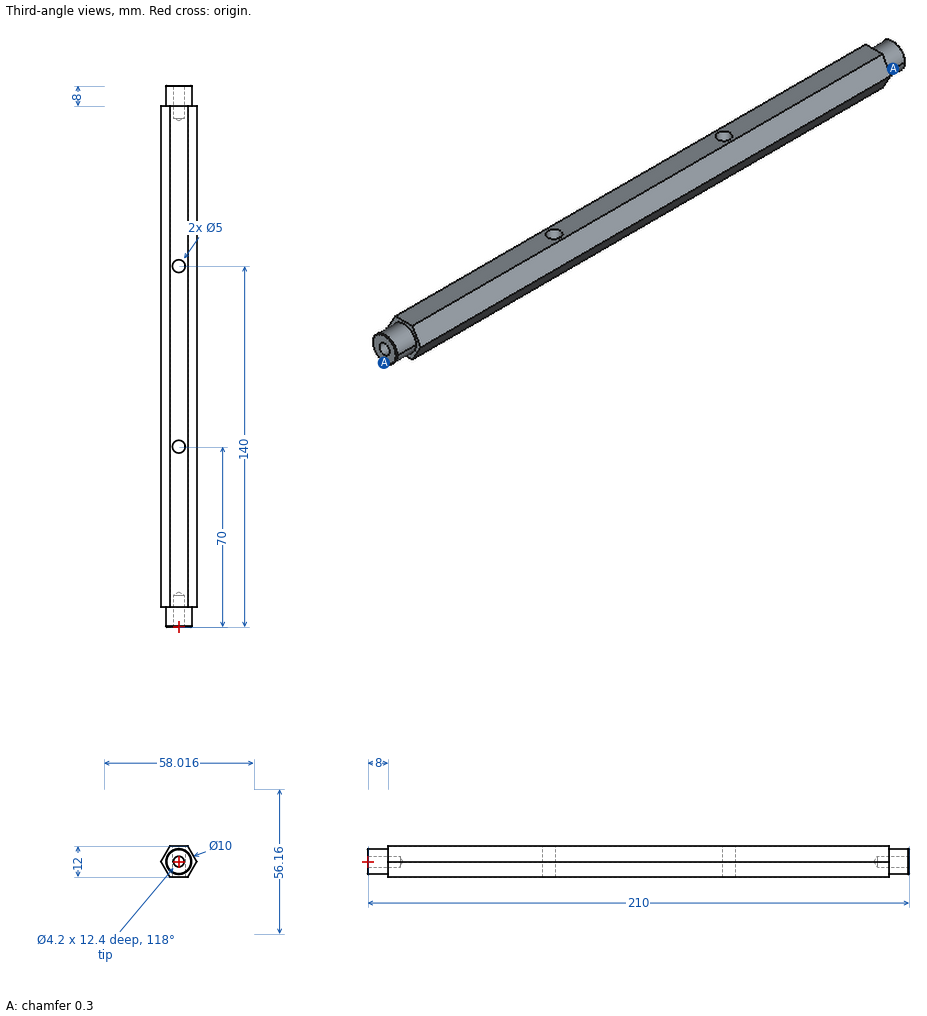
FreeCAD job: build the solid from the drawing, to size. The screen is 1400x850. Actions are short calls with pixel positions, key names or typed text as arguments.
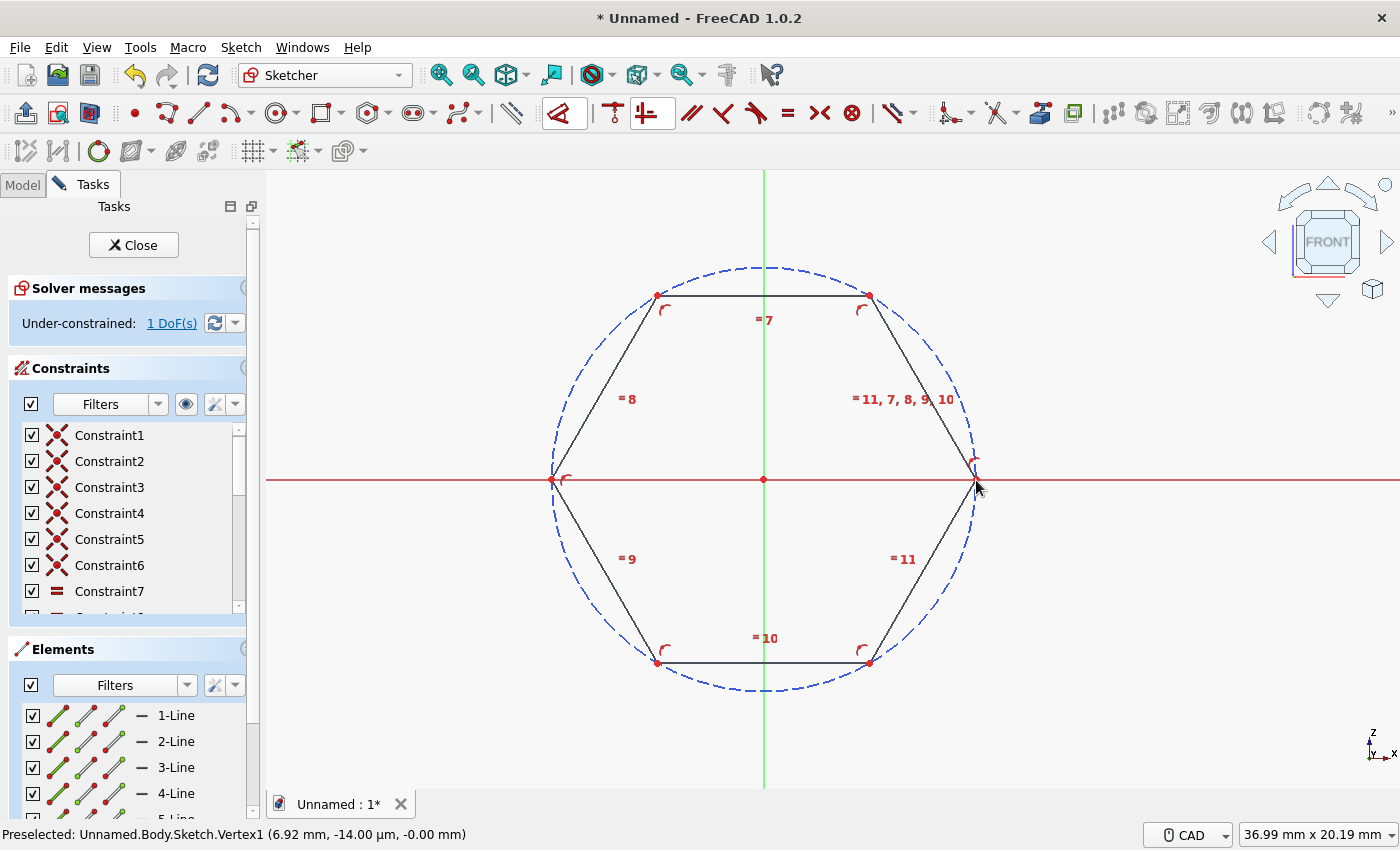
click(658, 663)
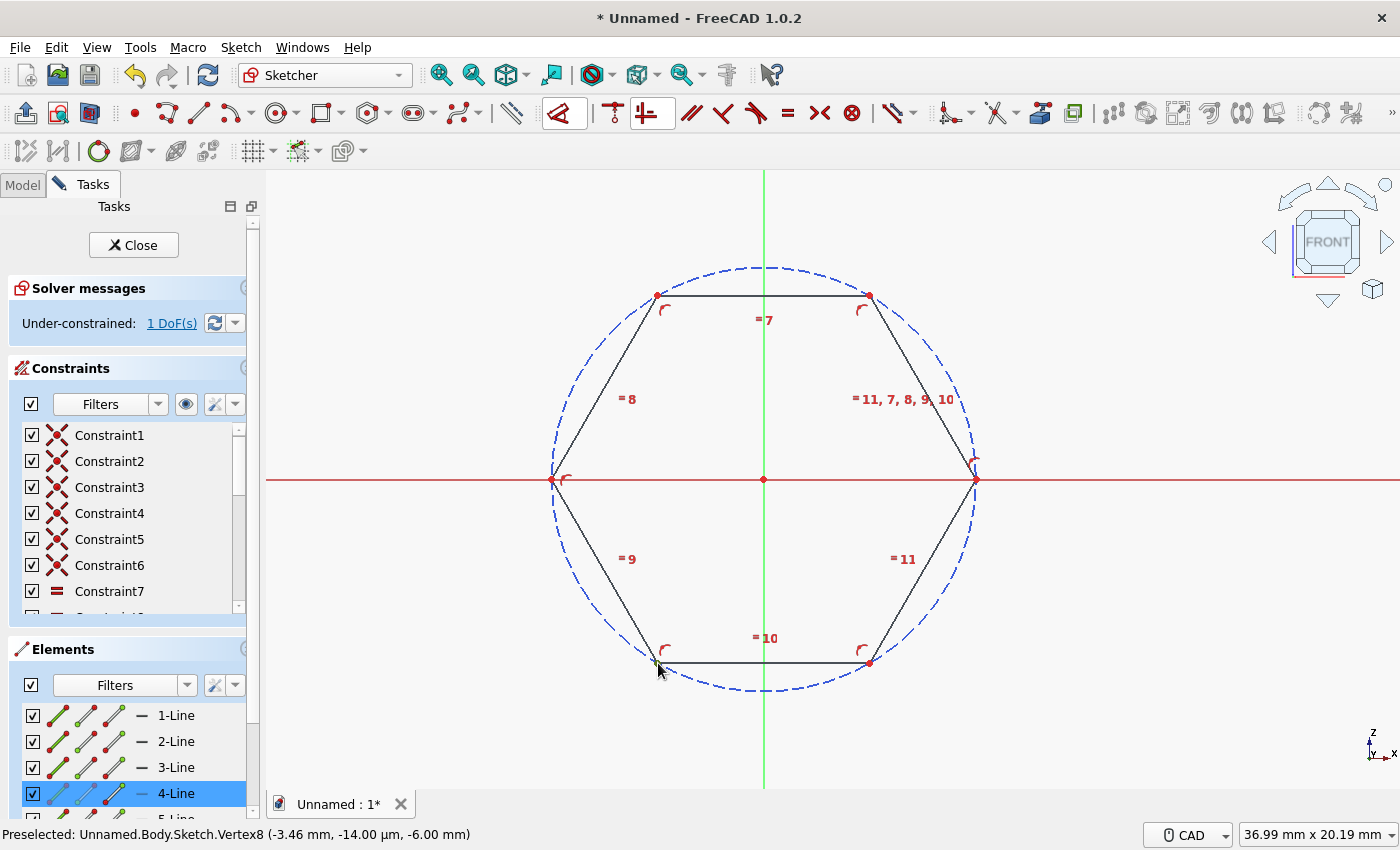
click(870, 296)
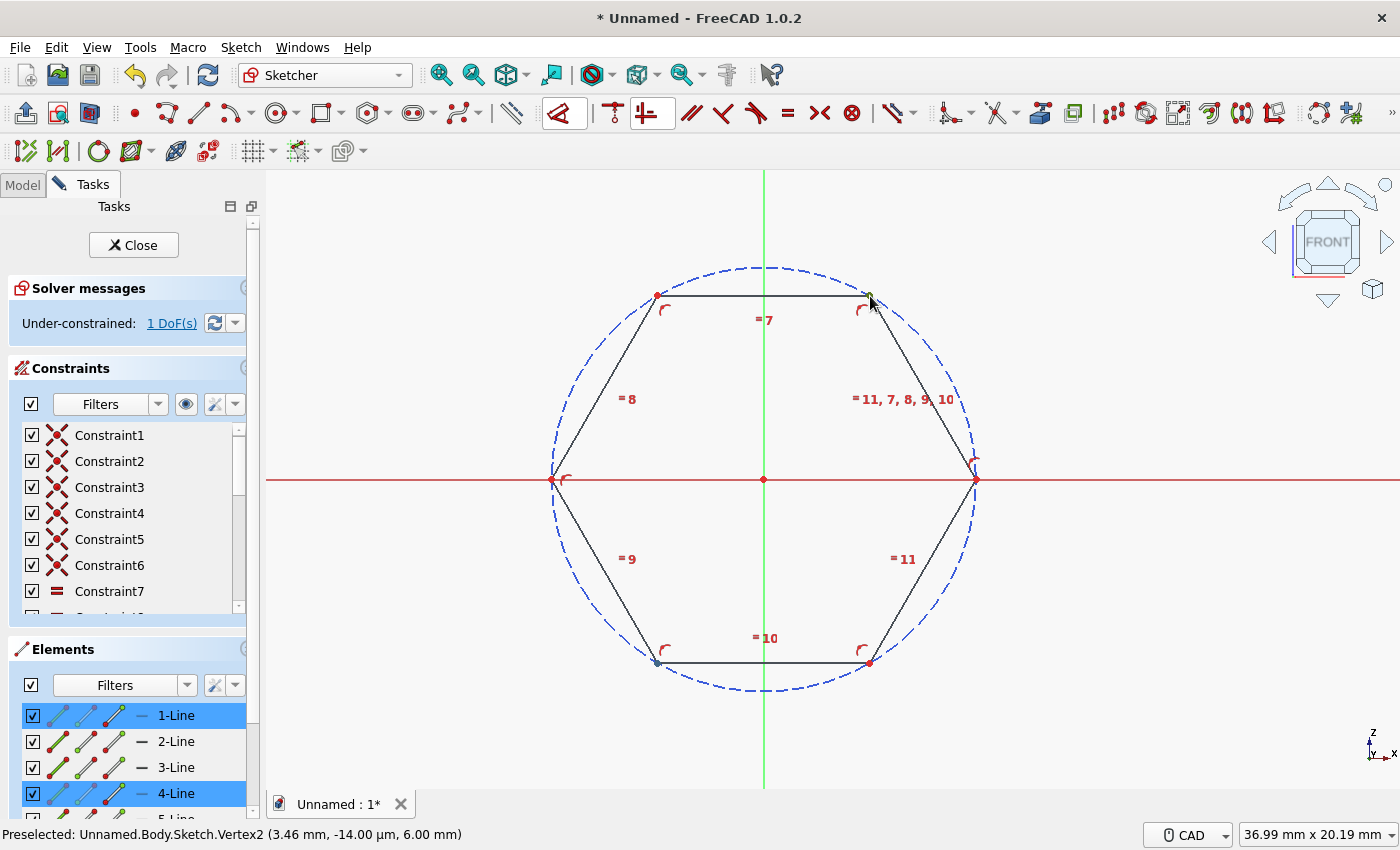
key(i)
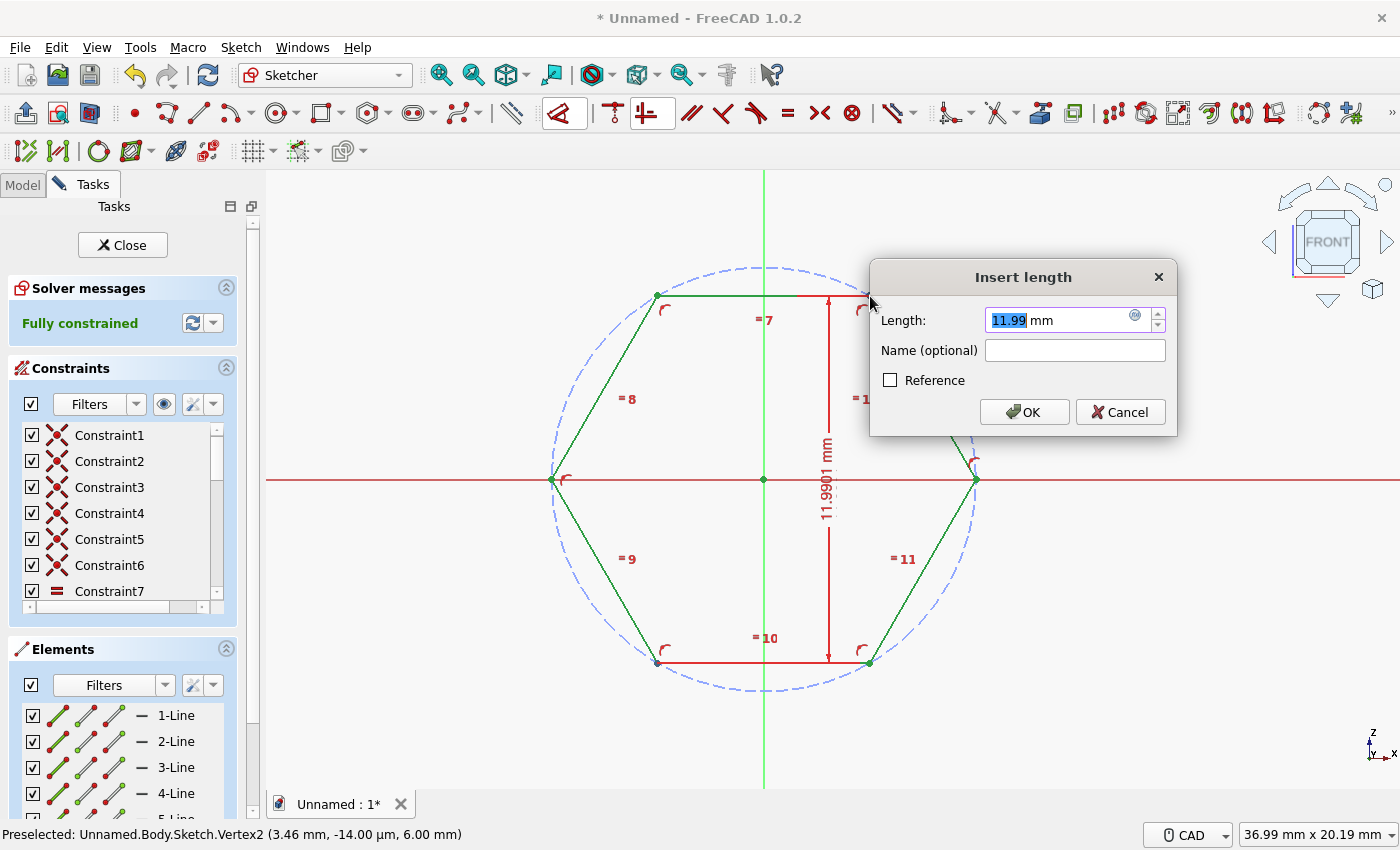
text(12)
key(Return)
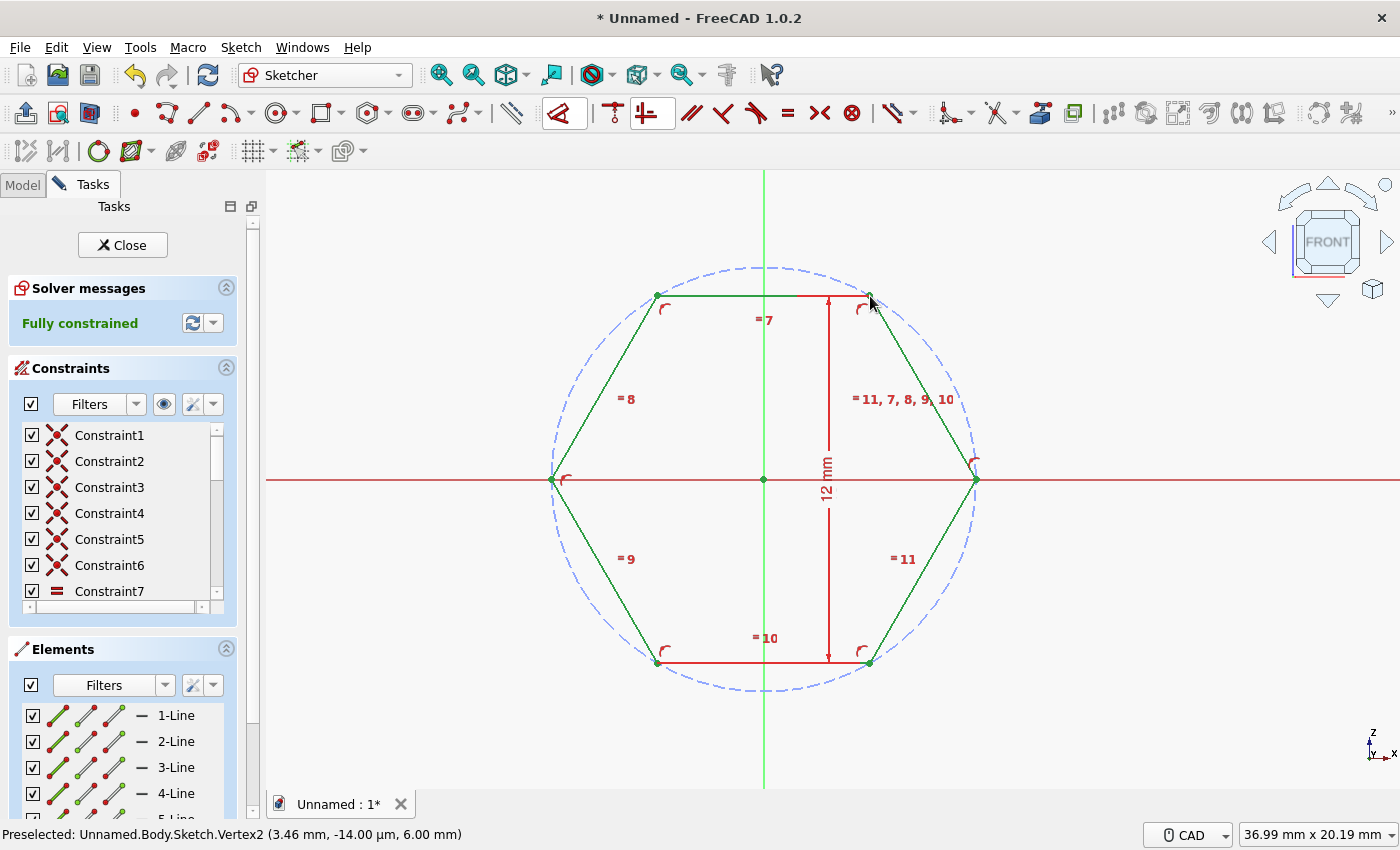
click(123, 245)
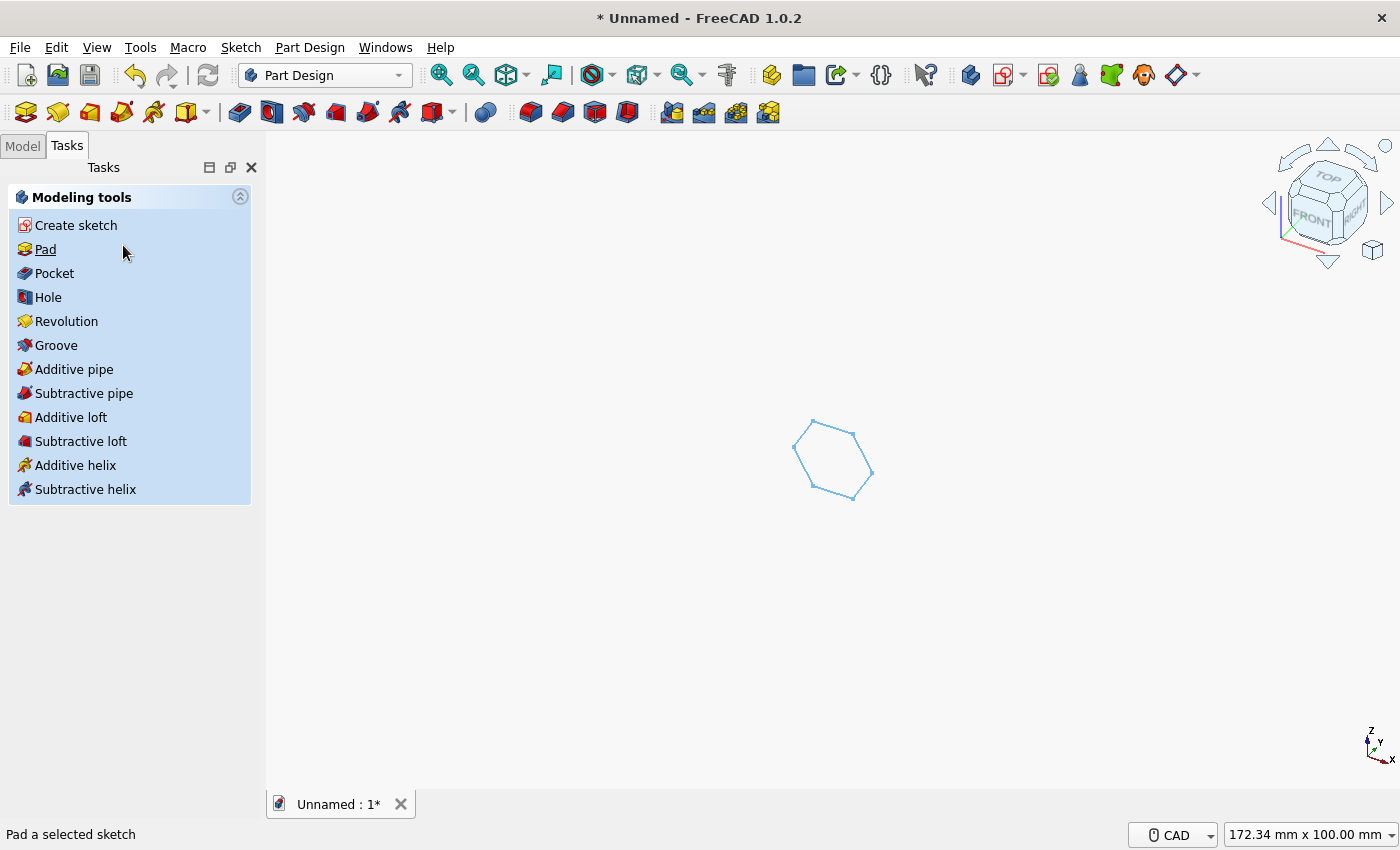
click(26, 112)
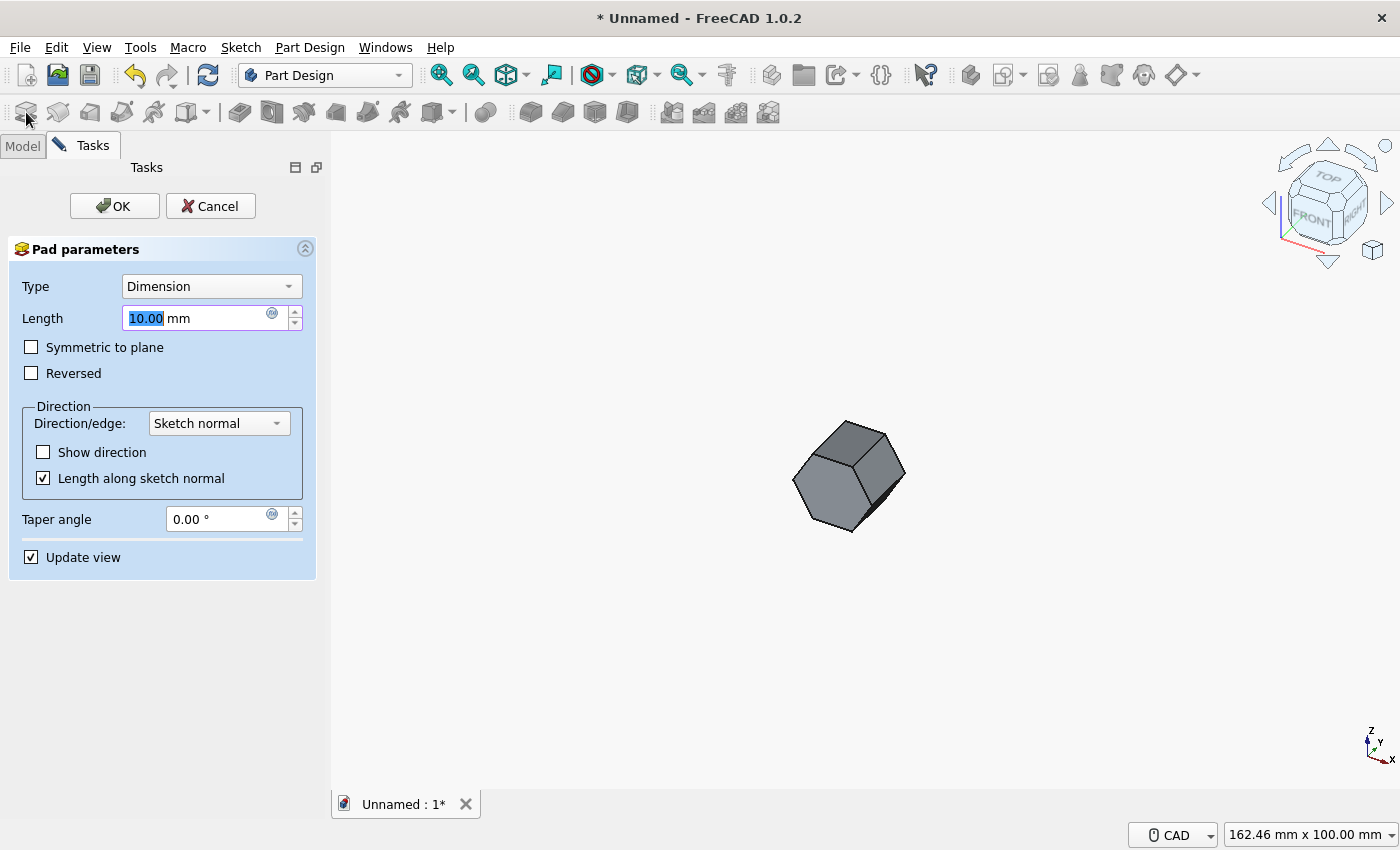
text(210)
key(Tab)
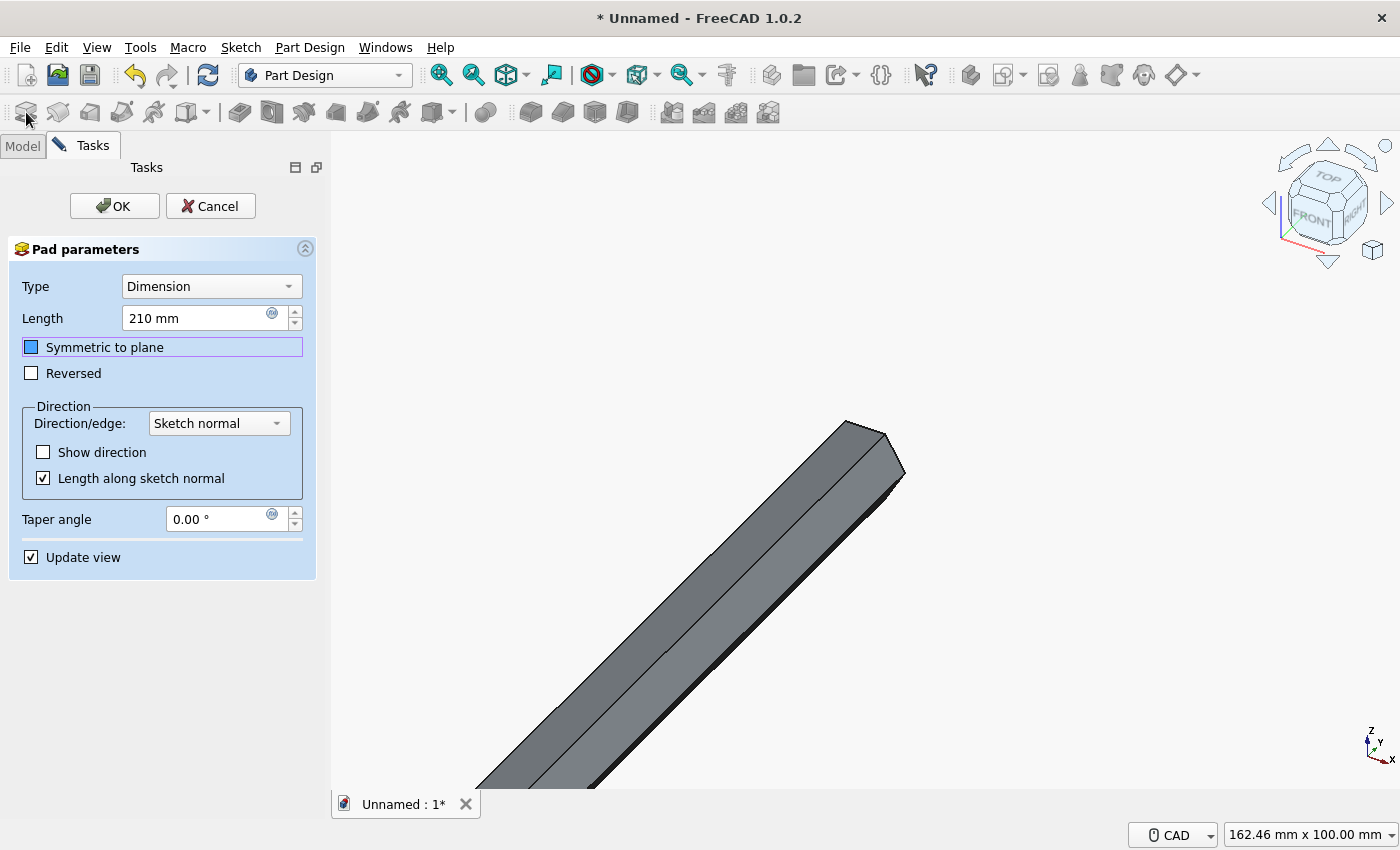
click(30, 373)